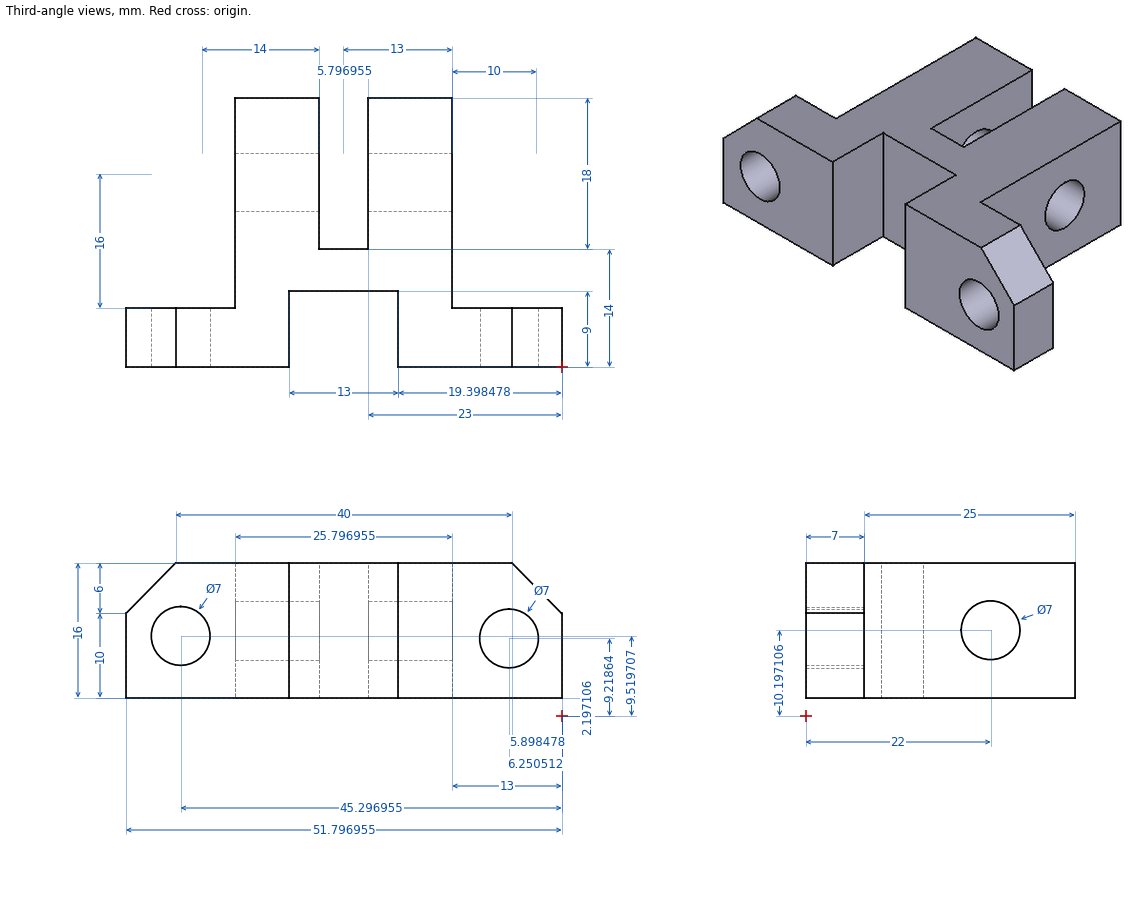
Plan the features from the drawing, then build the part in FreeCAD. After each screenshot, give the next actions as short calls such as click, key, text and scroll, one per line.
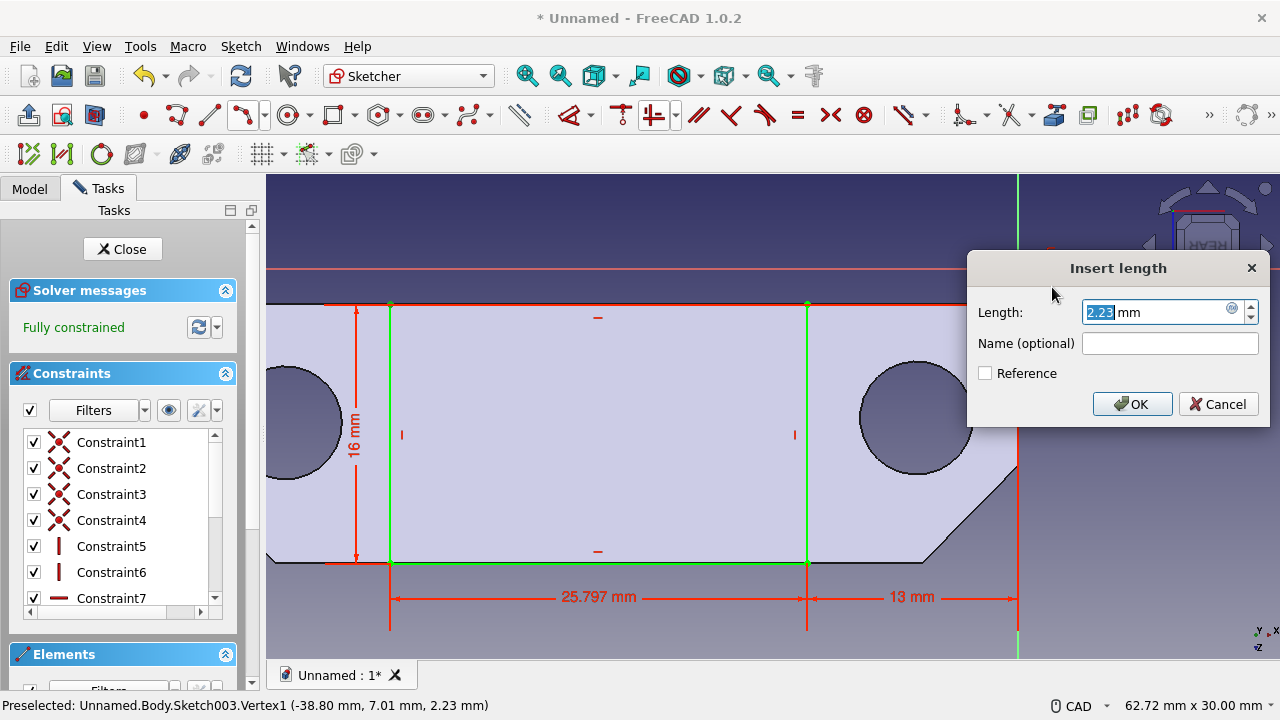
text(2.197106)
key(Return)
key(Escape)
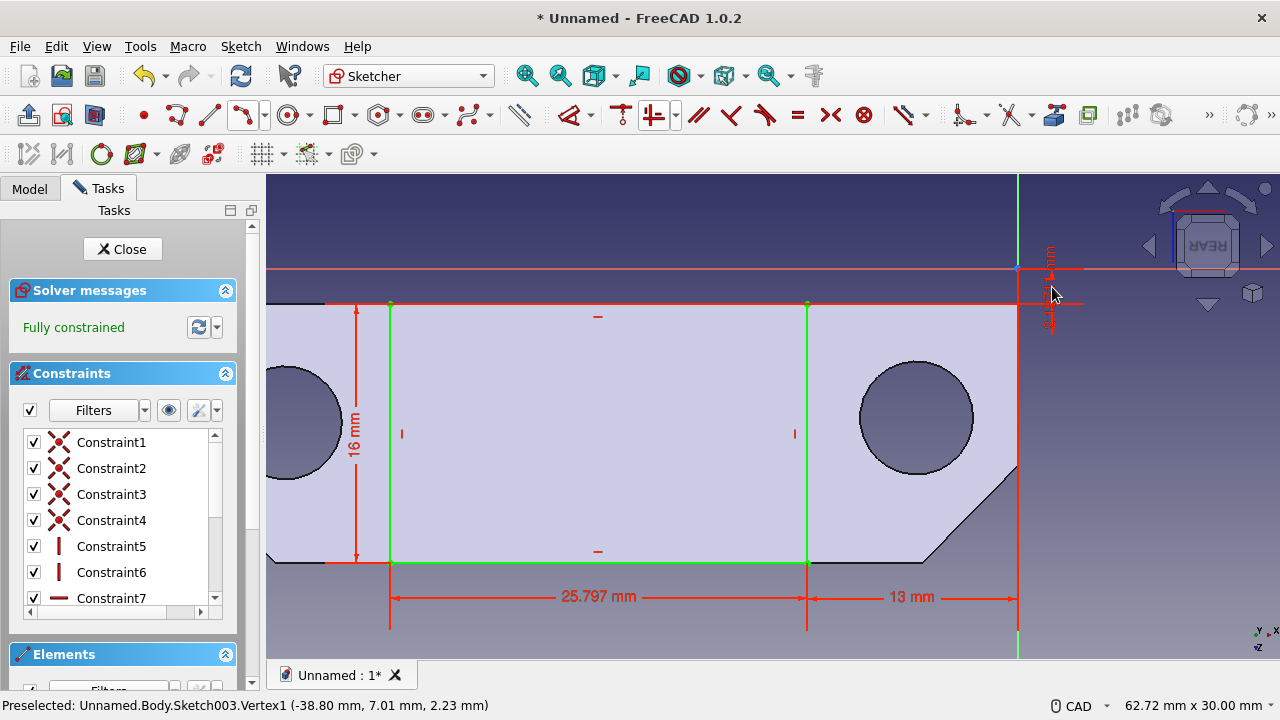
click(123, 249)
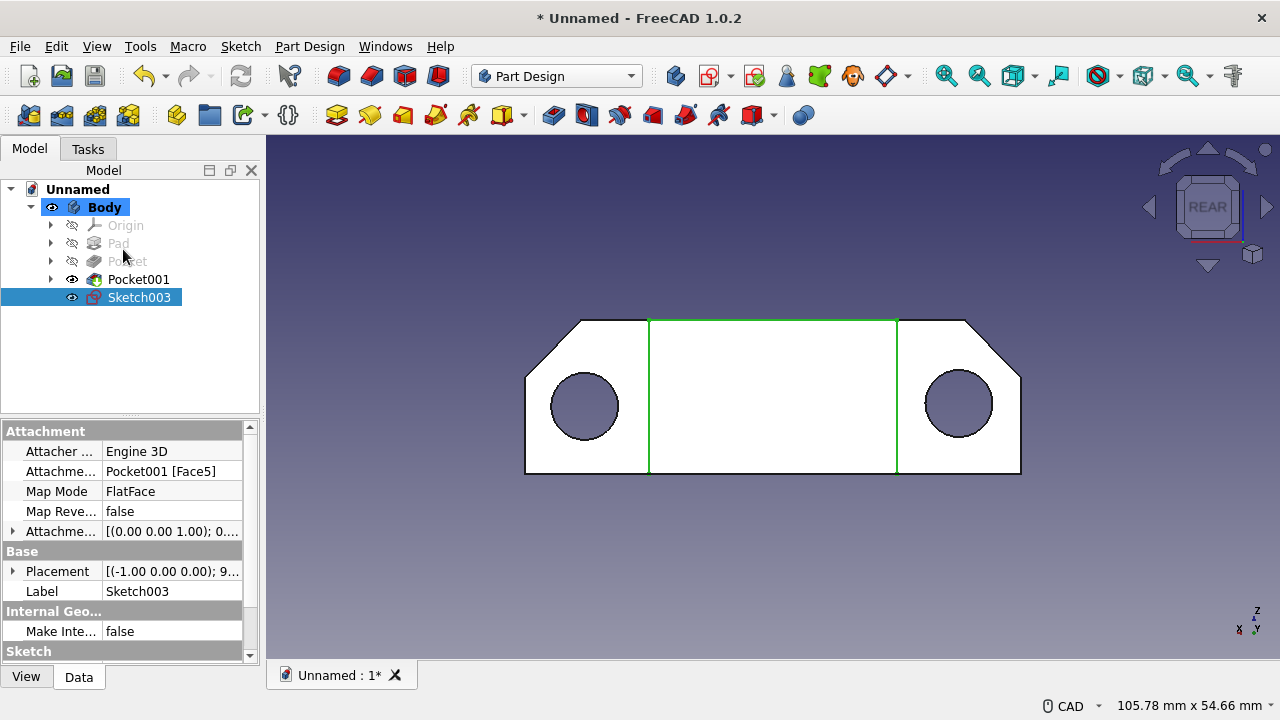
click(337, 116)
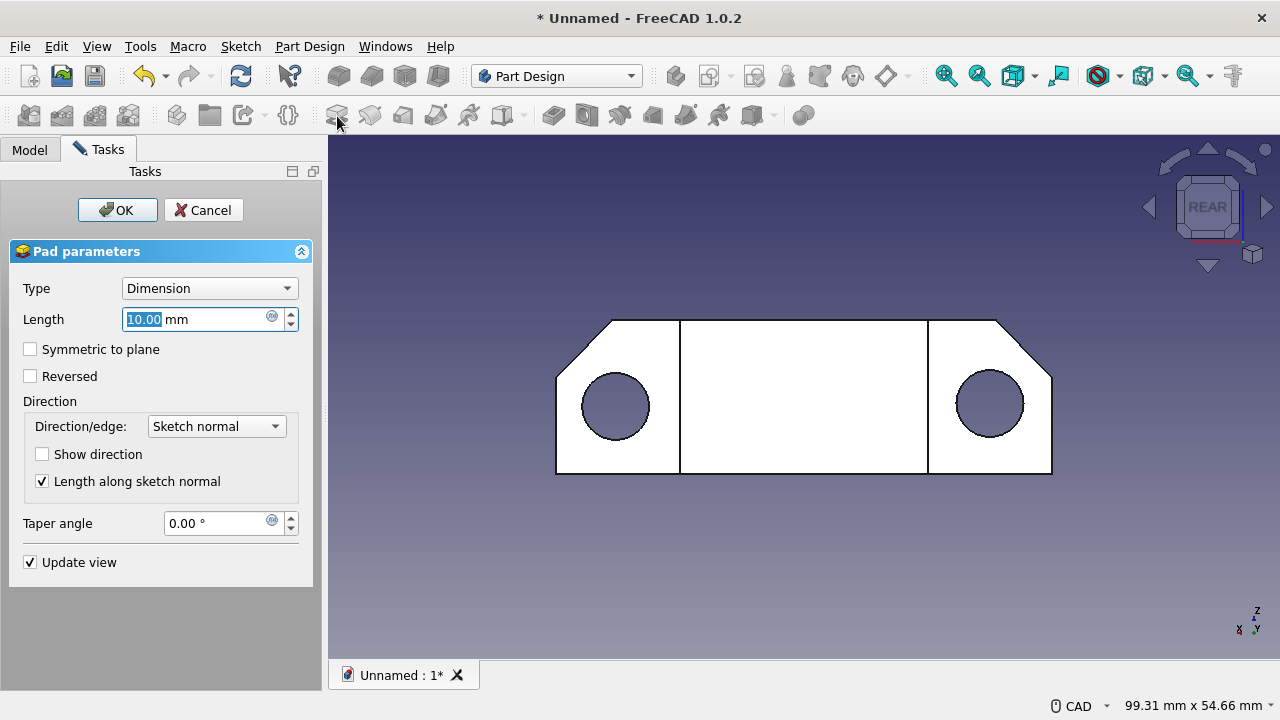
text(25)
key(Tab)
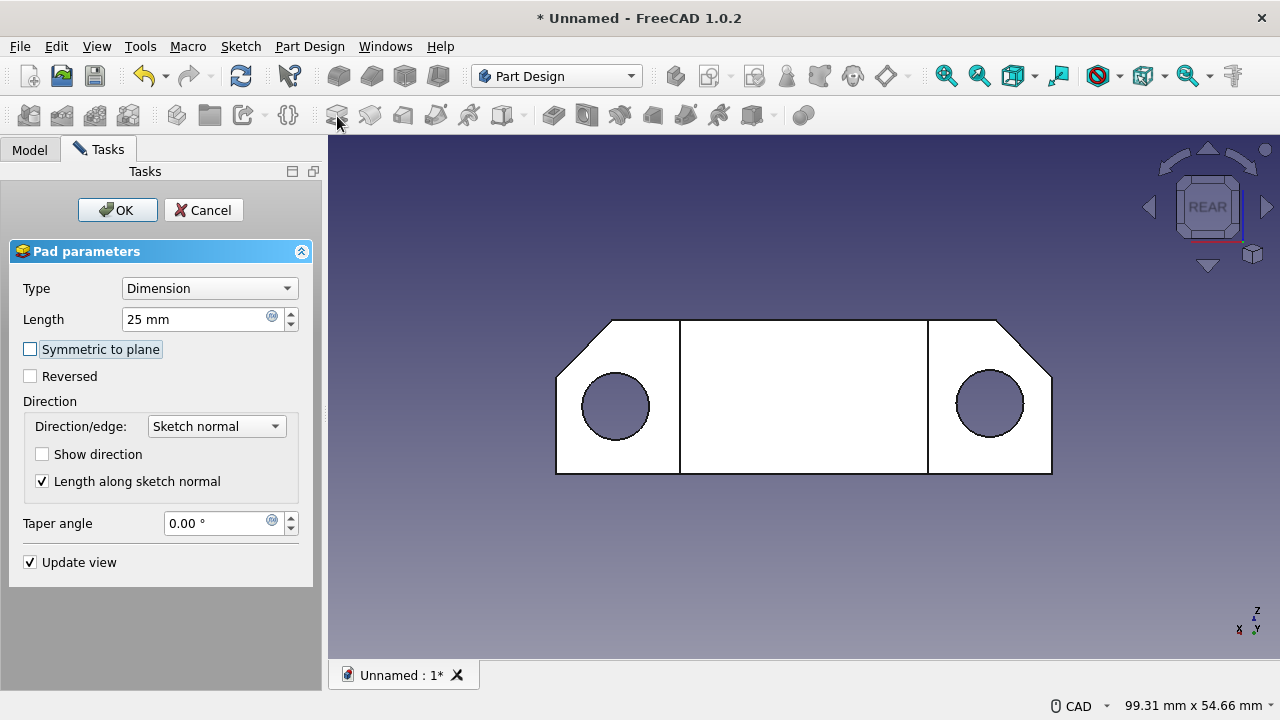
click(118, 210)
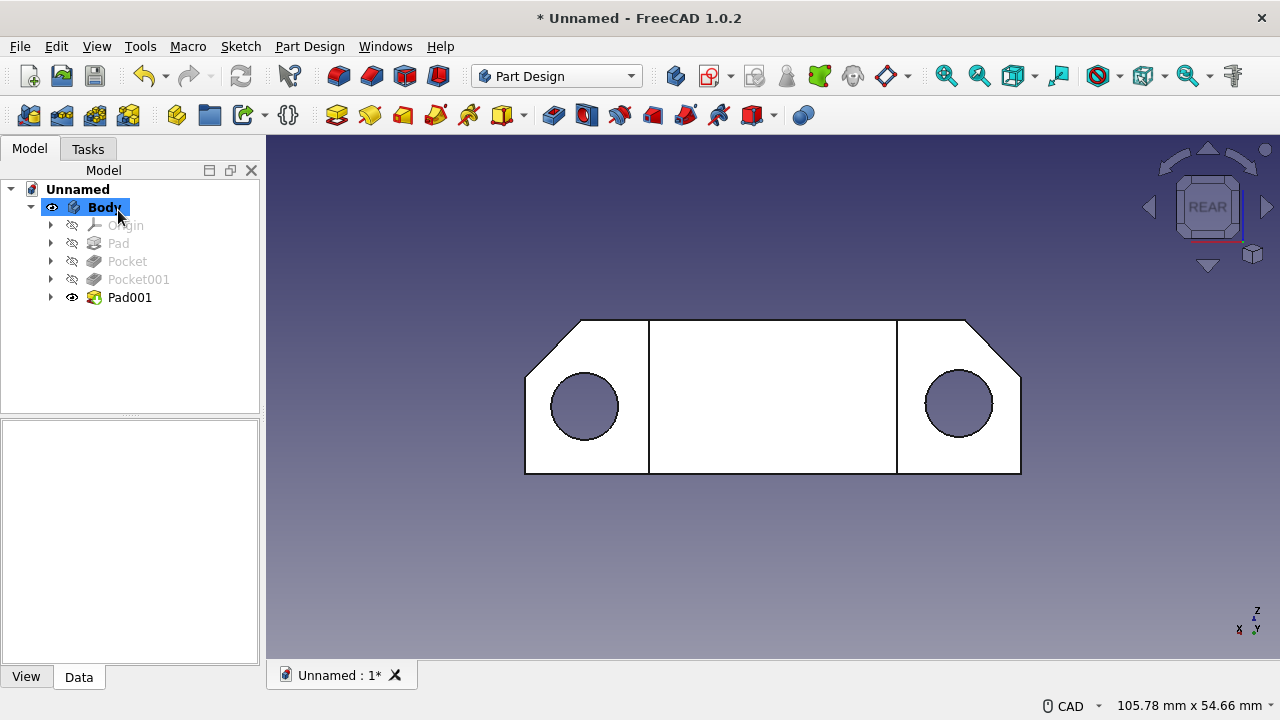
key(0)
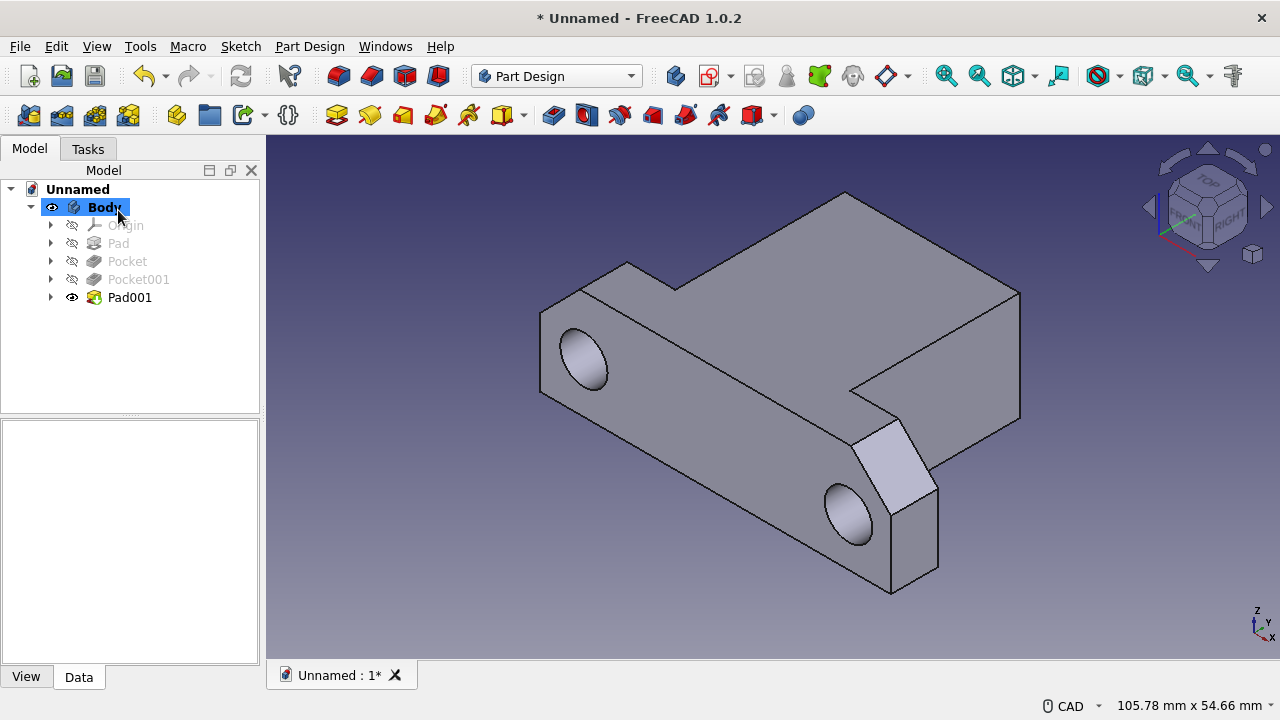
click(824, 304)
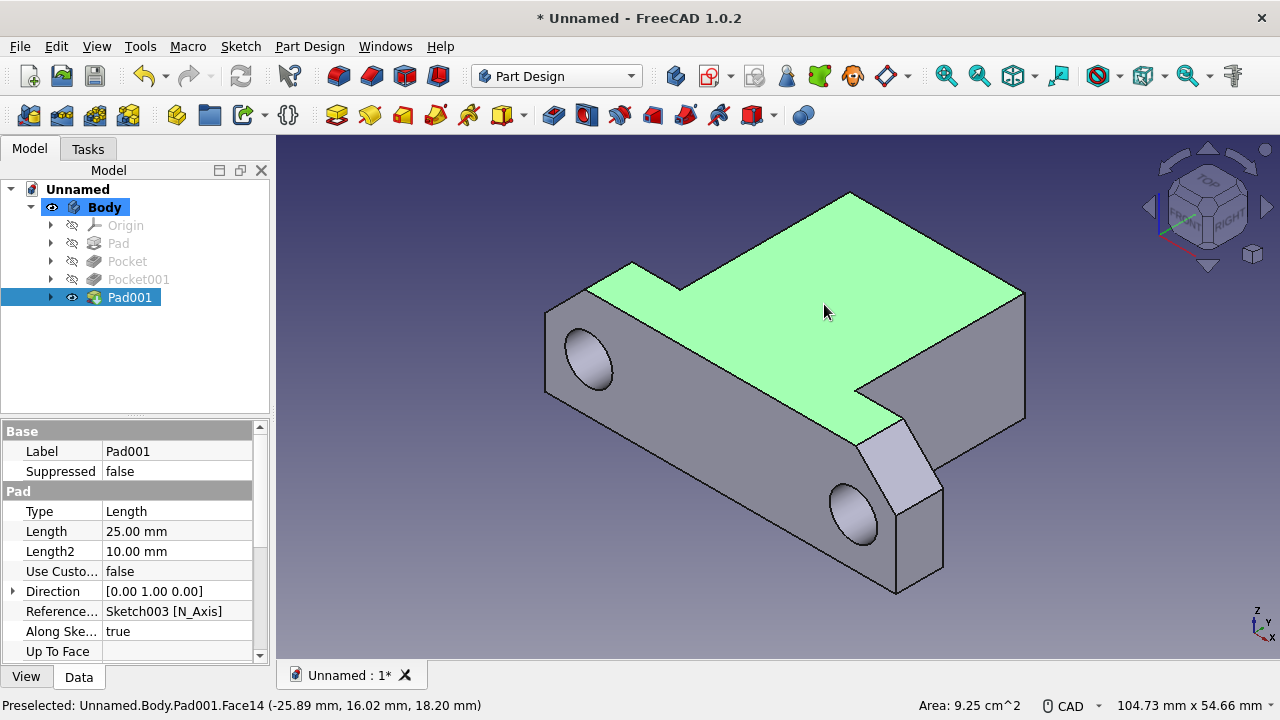
click(708, 76)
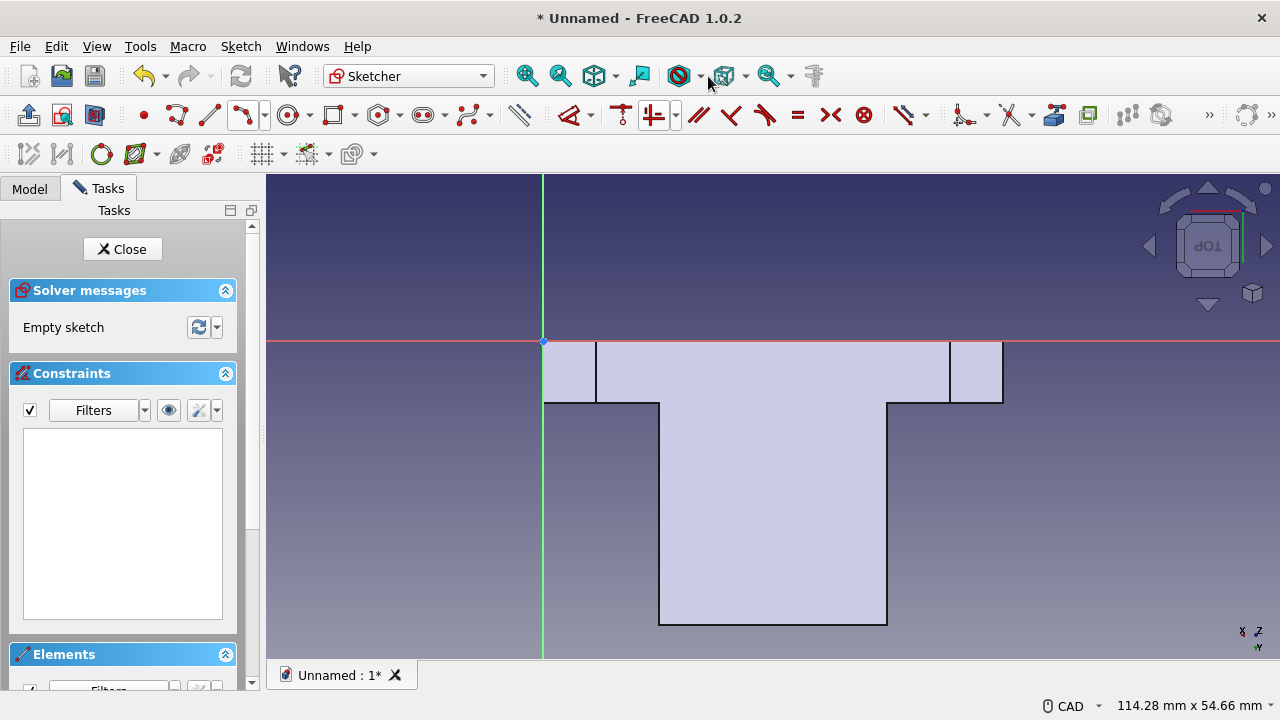
scroll(856, 202, down, 1)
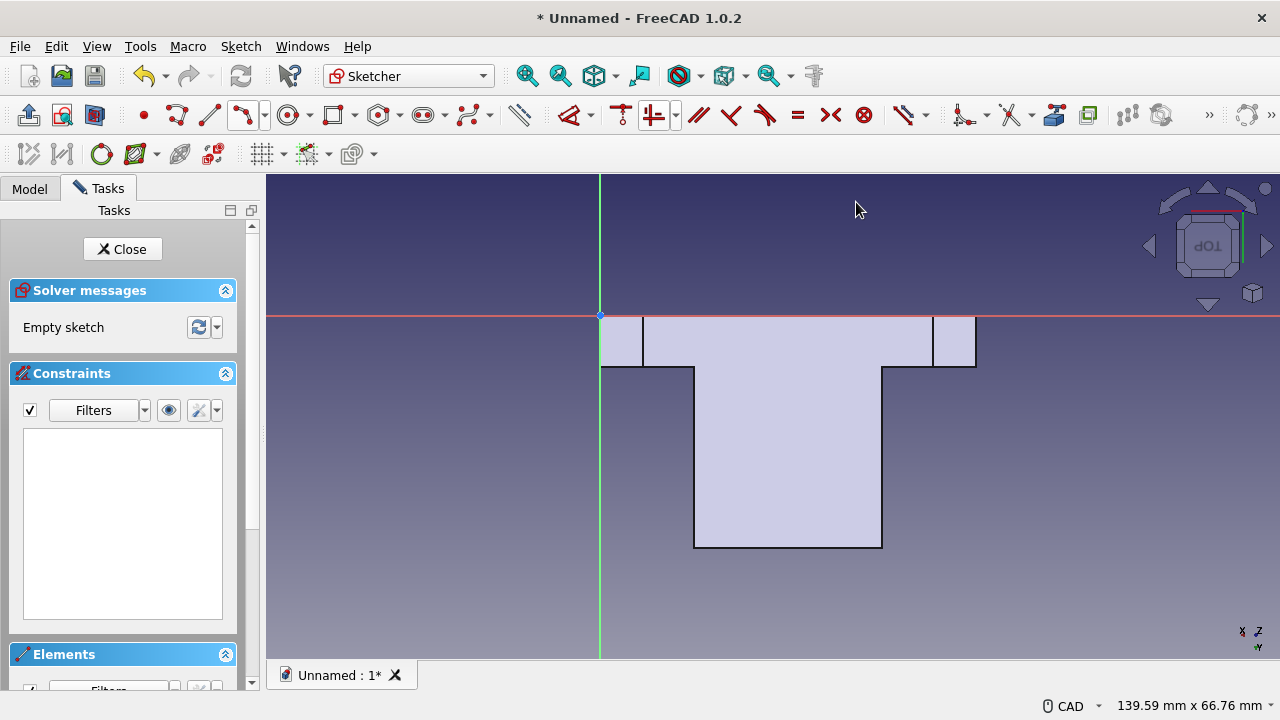
key(g)
key(r)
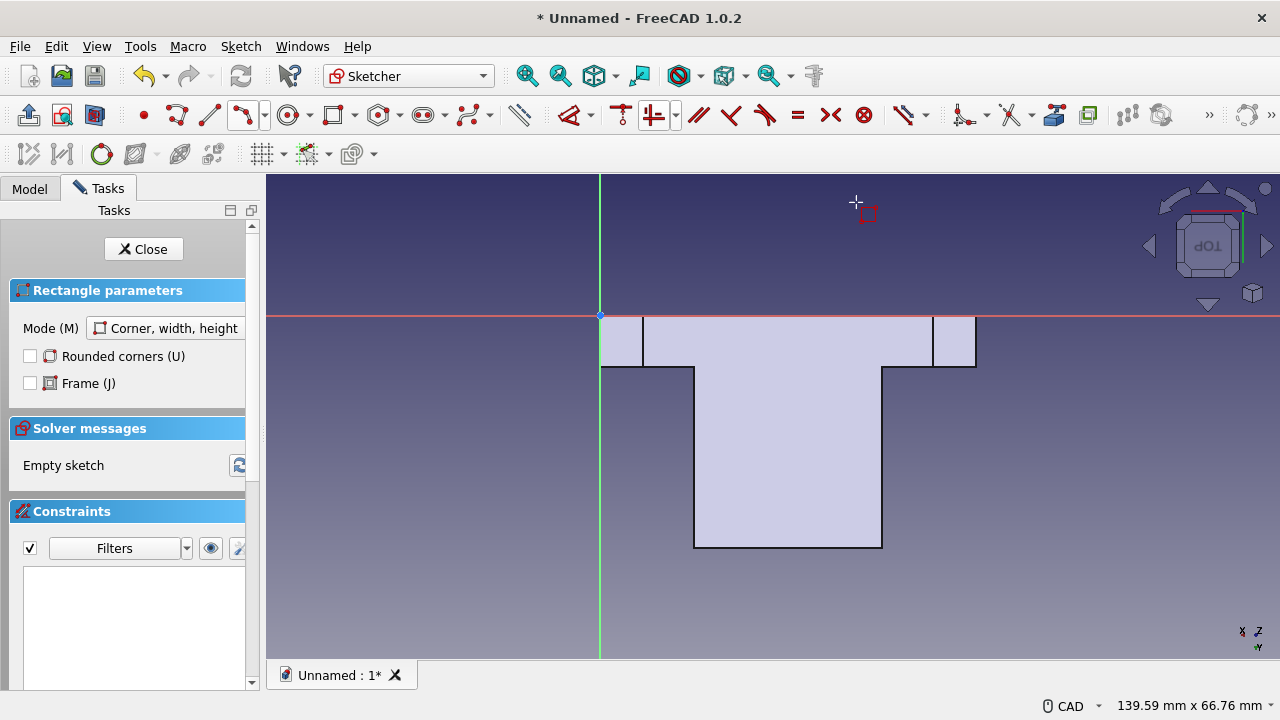
click(767, 418)
click(809, 548)
key(Escape)